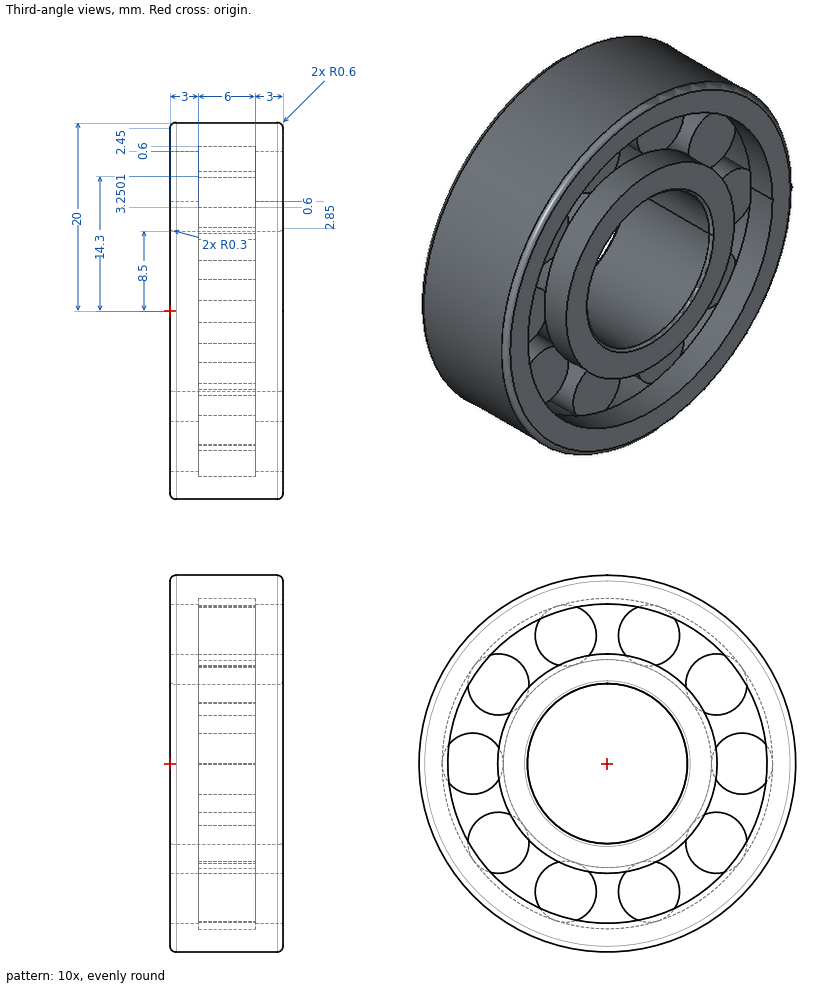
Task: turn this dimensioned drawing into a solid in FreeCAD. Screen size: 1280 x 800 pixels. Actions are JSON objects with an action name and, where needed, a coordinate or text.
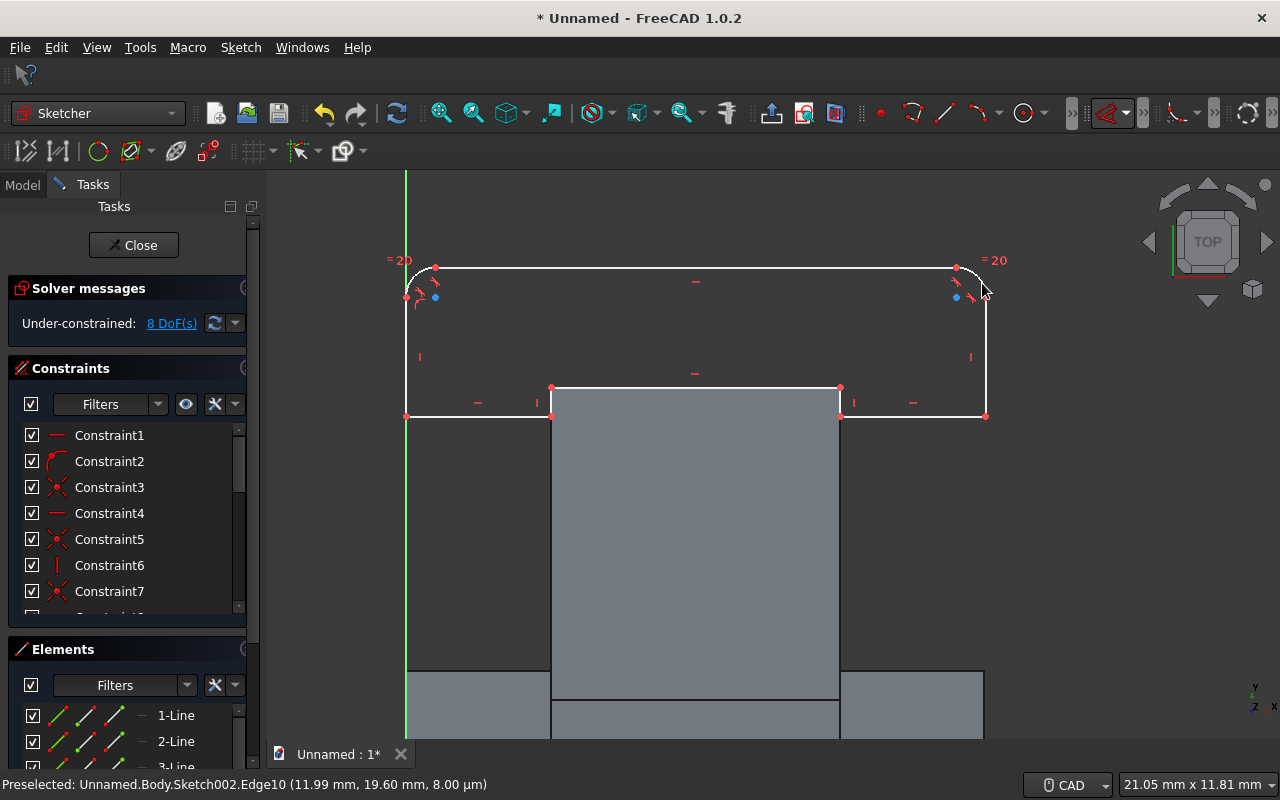
{"action": "scroll", "coordinate": [422, 271], "scroll_direction": "up", "scroll_amount": 2}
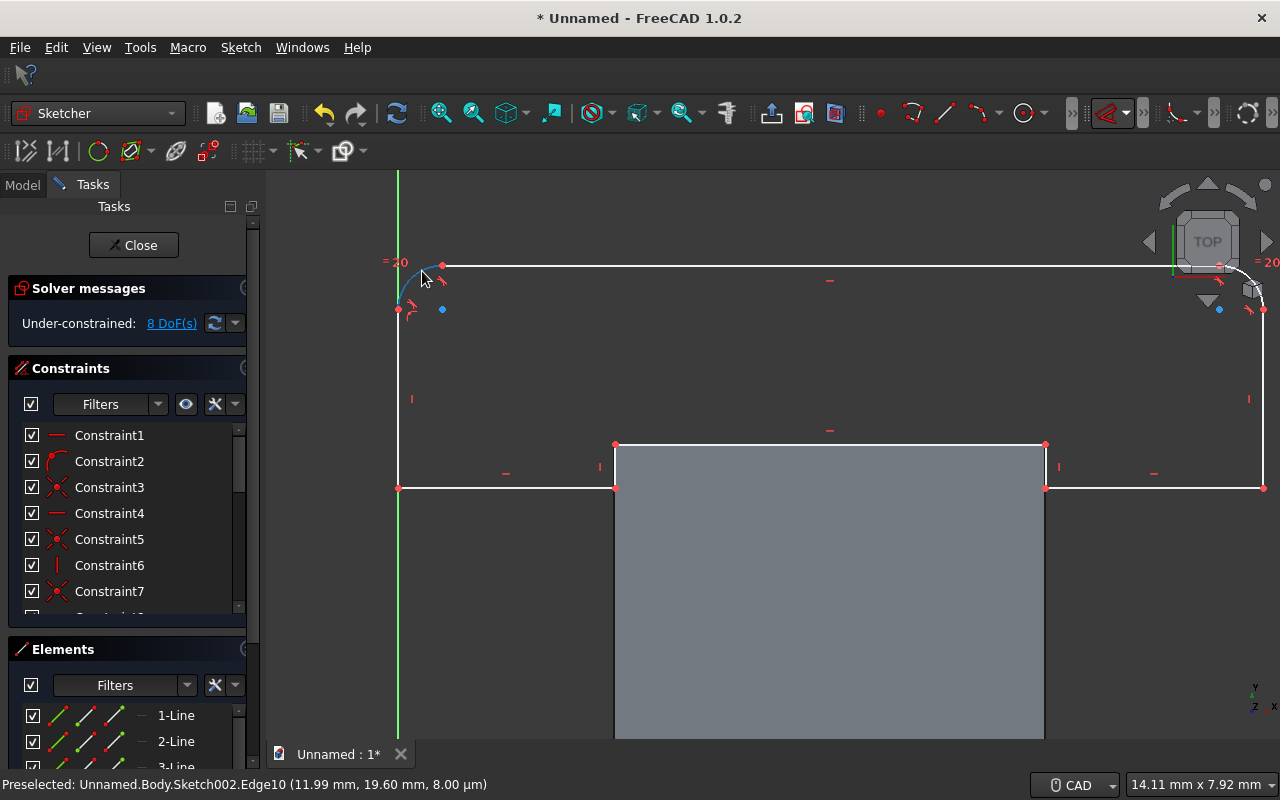
{"action": "left_click", "coordinate": [422, 271]}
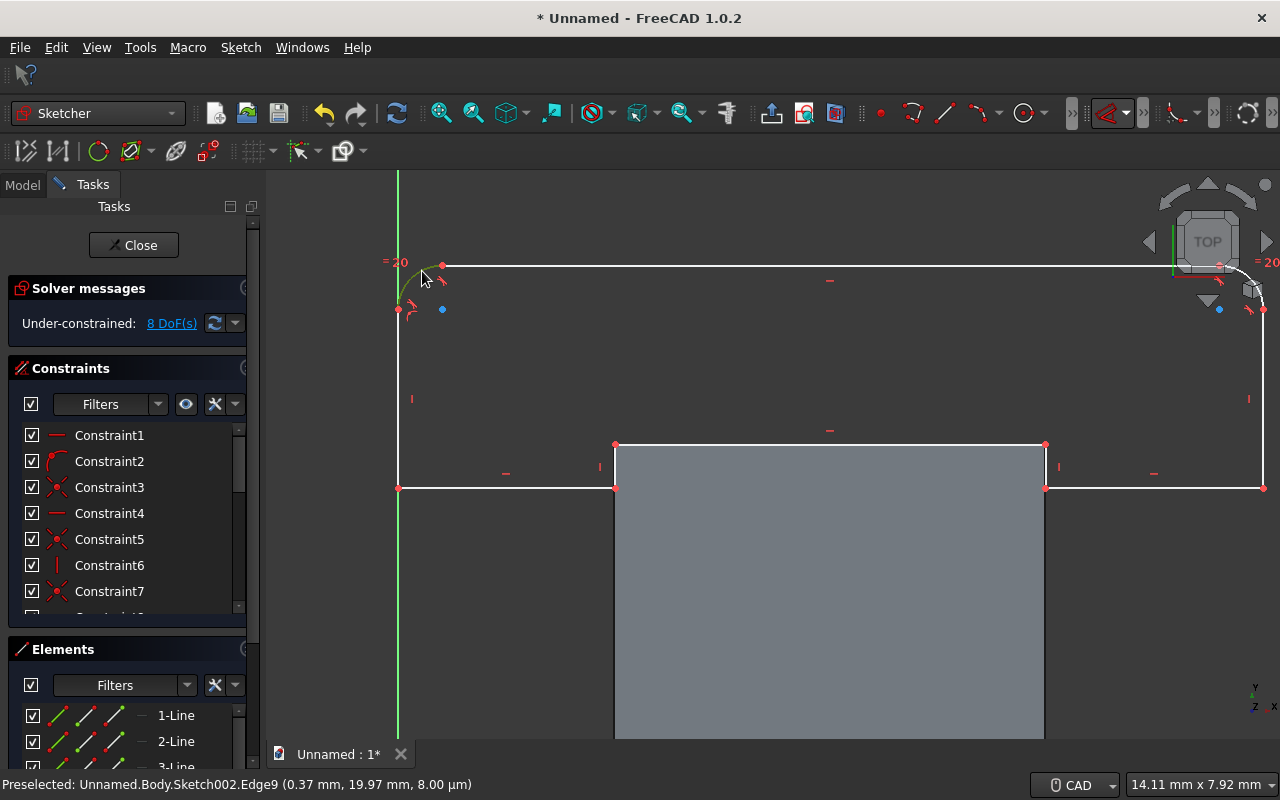
{"action": "key", "text": "k r"}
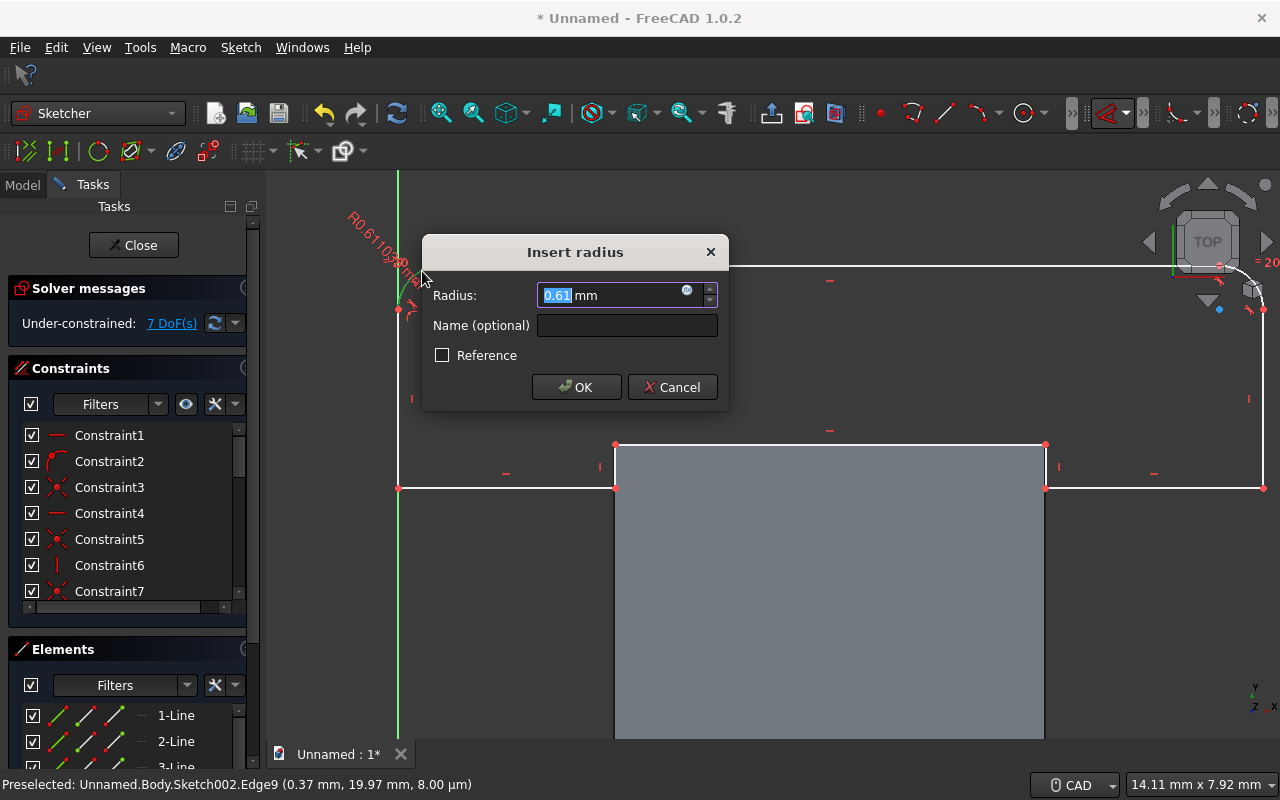
{"action": "type", "text": "0.6"}
{"action": "key", "text": "Return"}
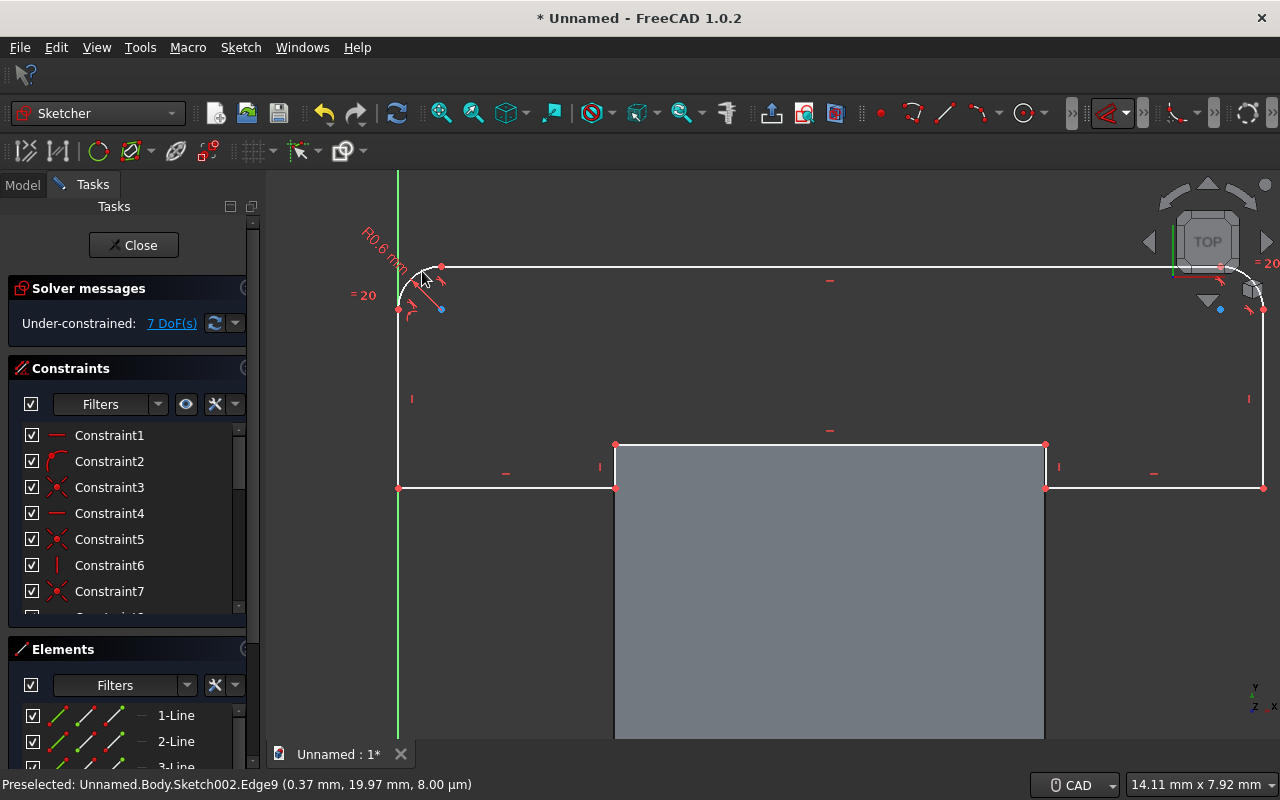
{"action": "scroll", "coordinate": [664, 281], "scroll_direction": "down", "scroll_amount": 7}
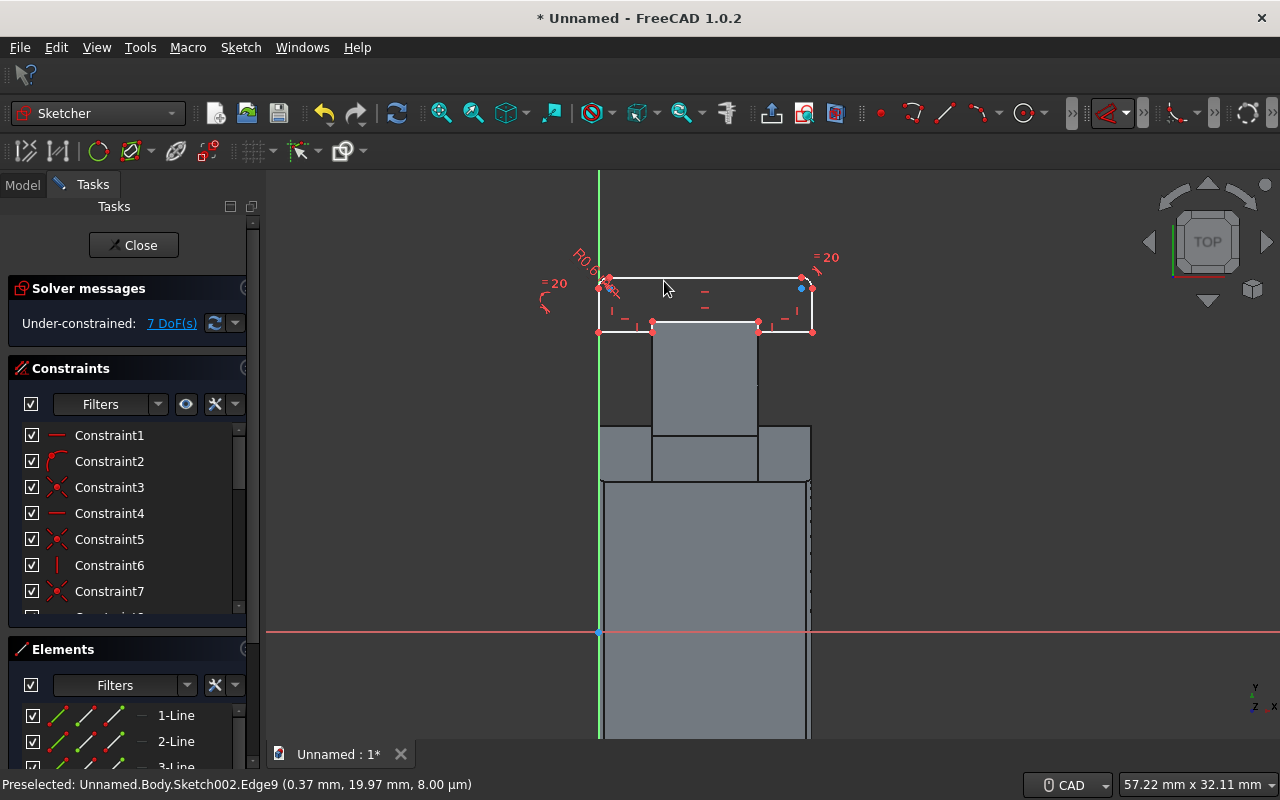
{"action": "left_click", "coordinate": [615, 332]}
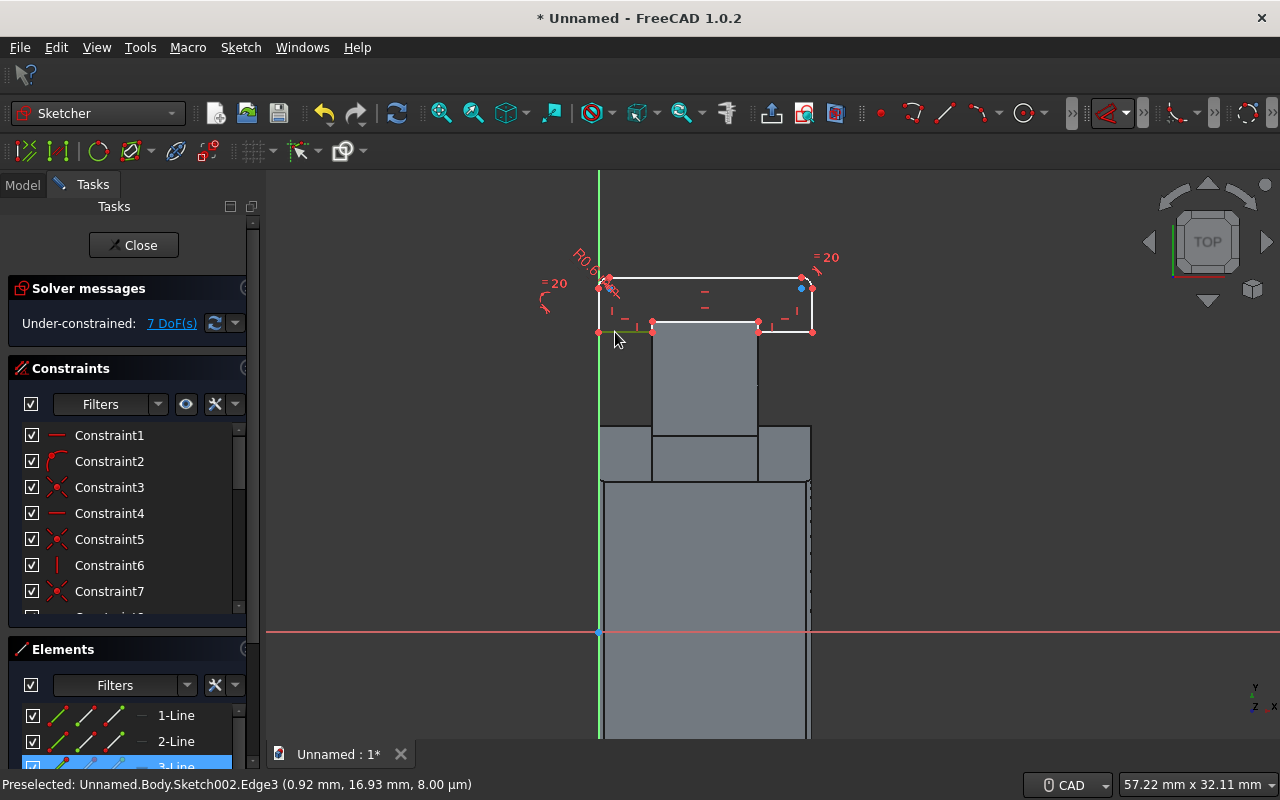
{"action": "key", "text": "l"}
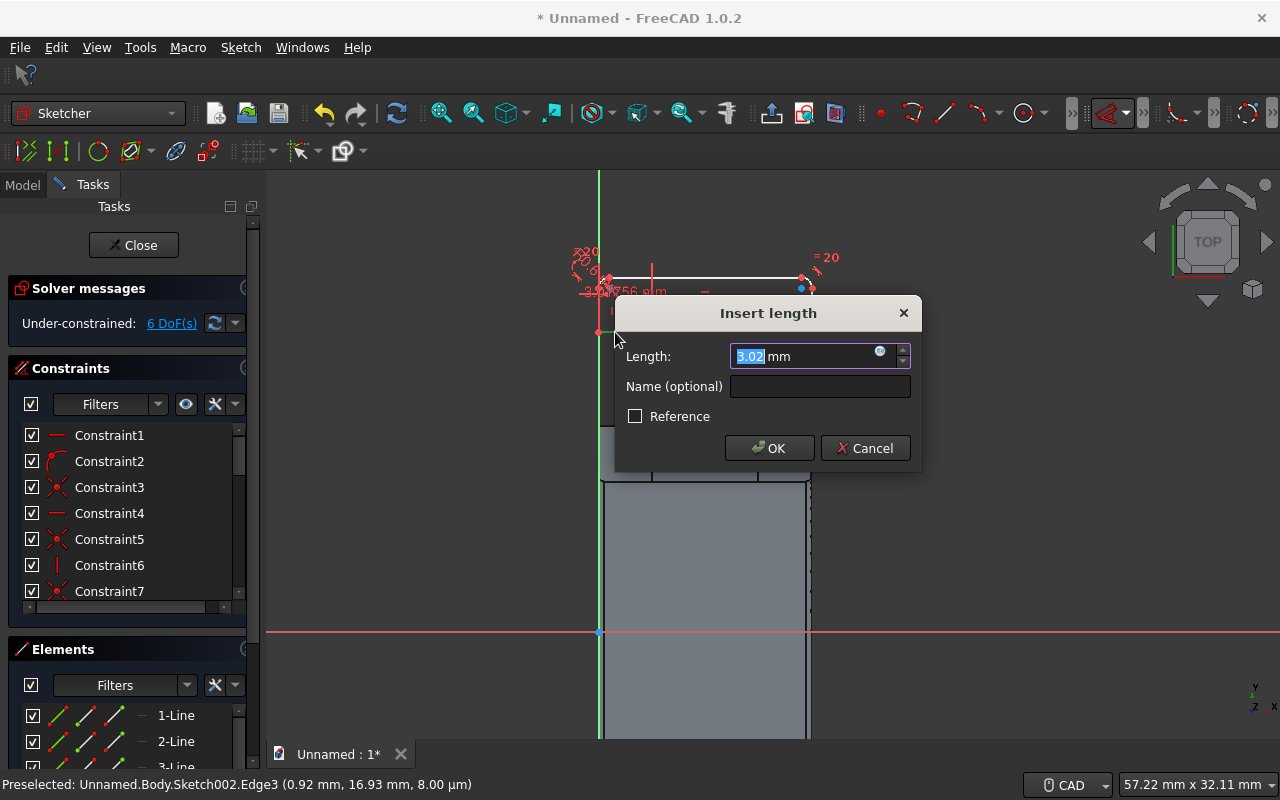
{"action": "type", "text": "3"}
{"action": "key", "text": "Return"}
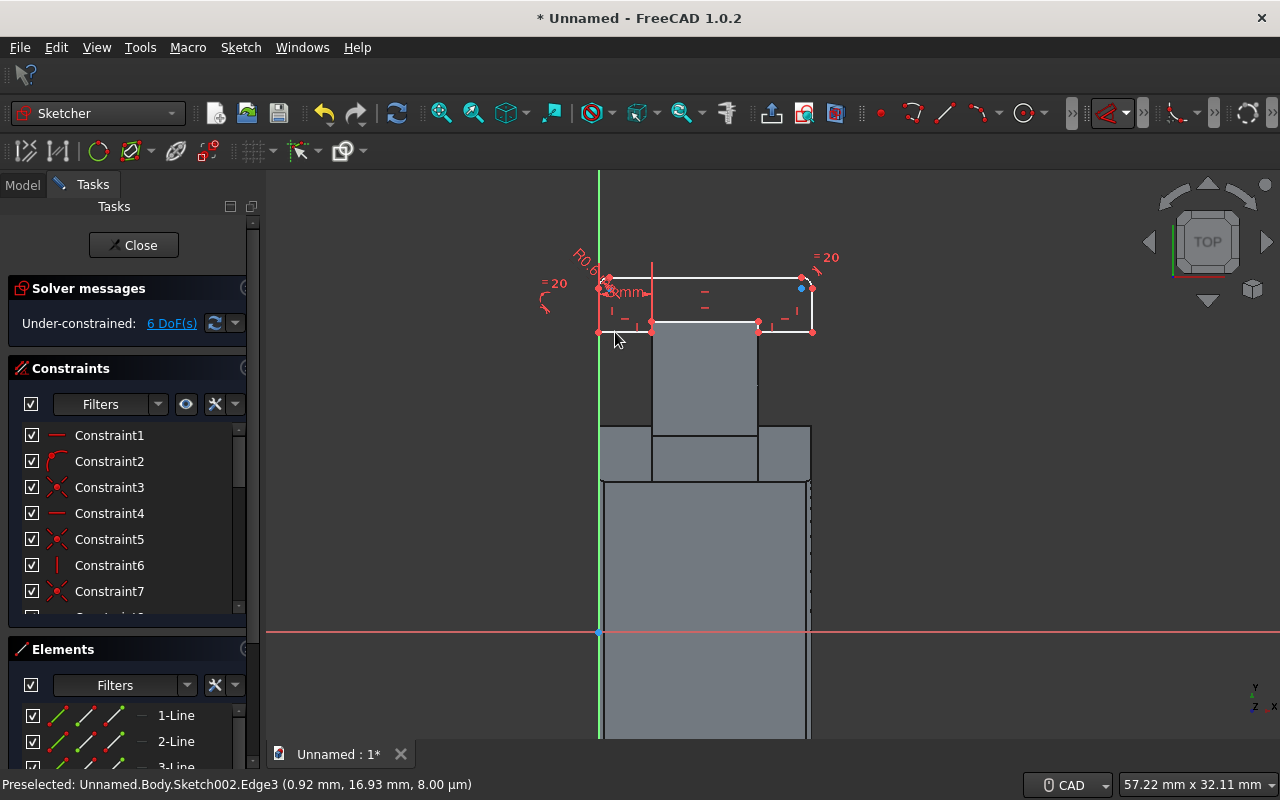
{"action": "left_click", "coordinate": [684, 322]}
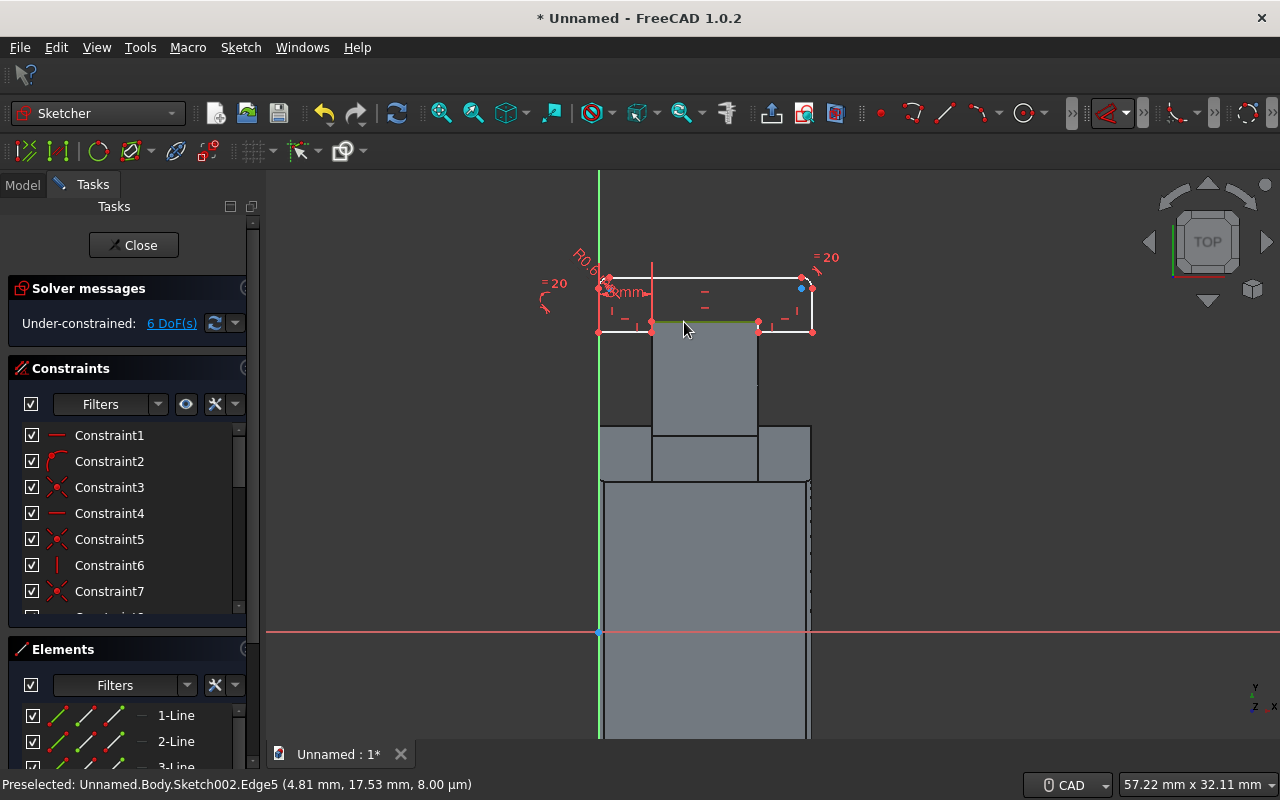
{"action": "left_click", "coordinate": [1128, 114]}